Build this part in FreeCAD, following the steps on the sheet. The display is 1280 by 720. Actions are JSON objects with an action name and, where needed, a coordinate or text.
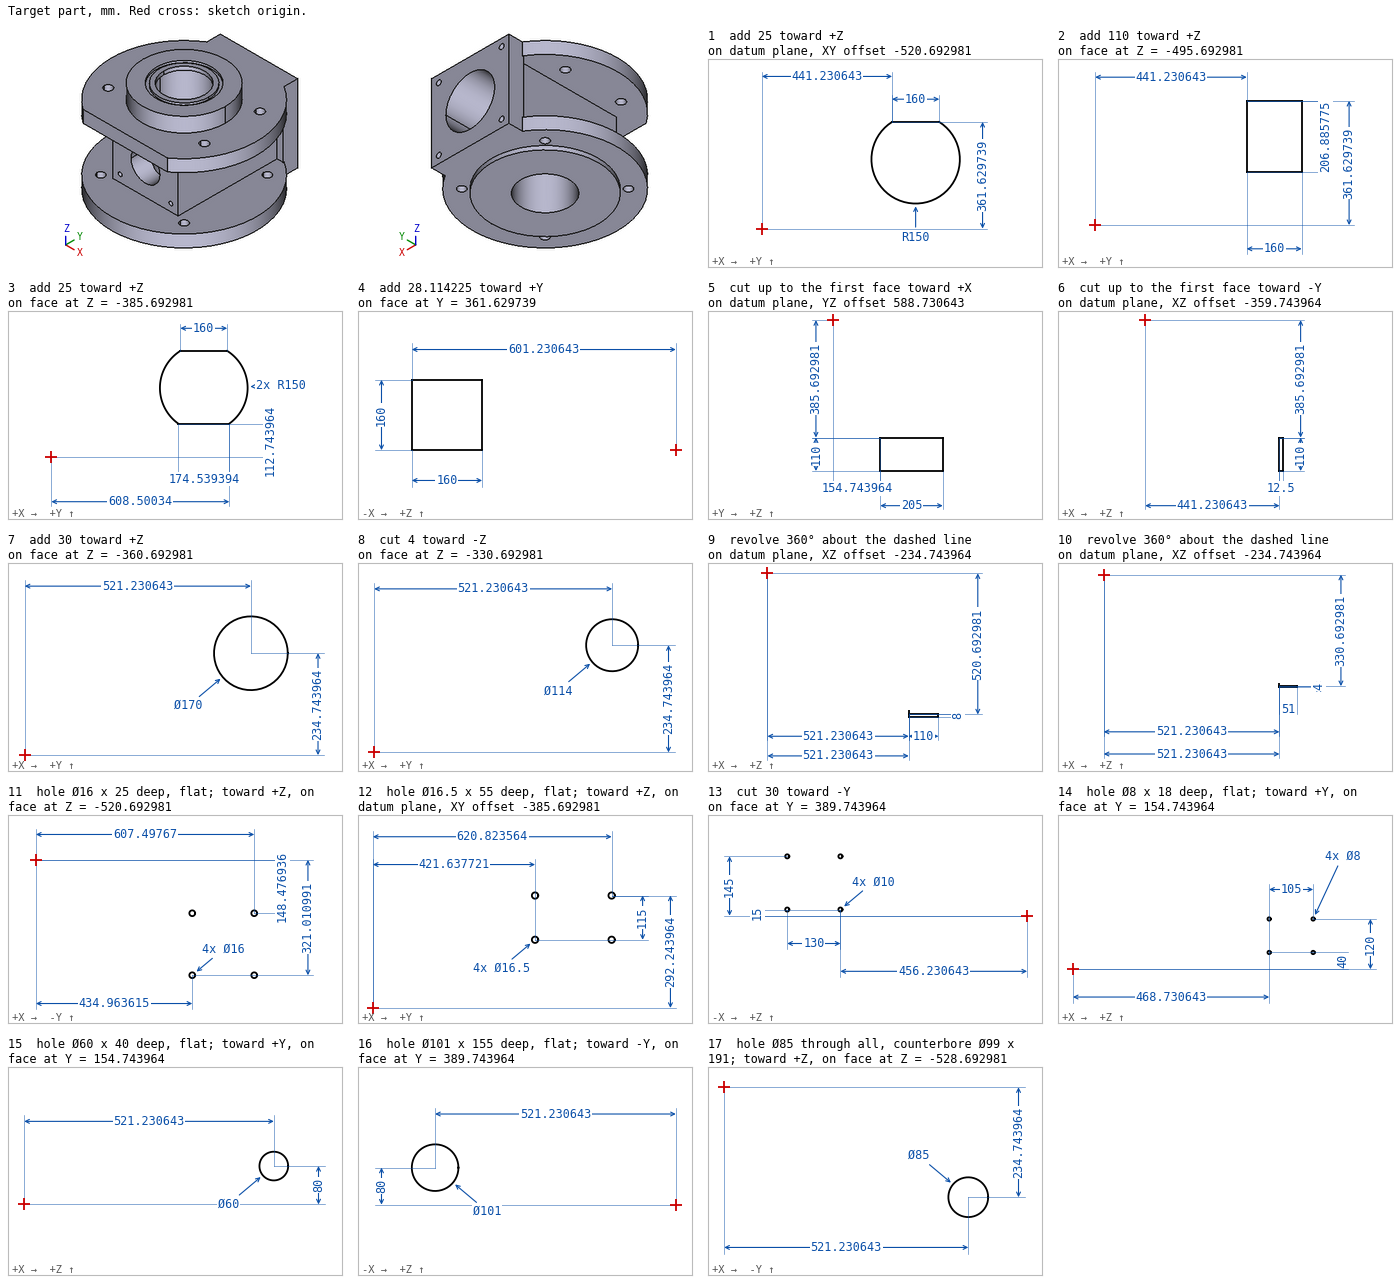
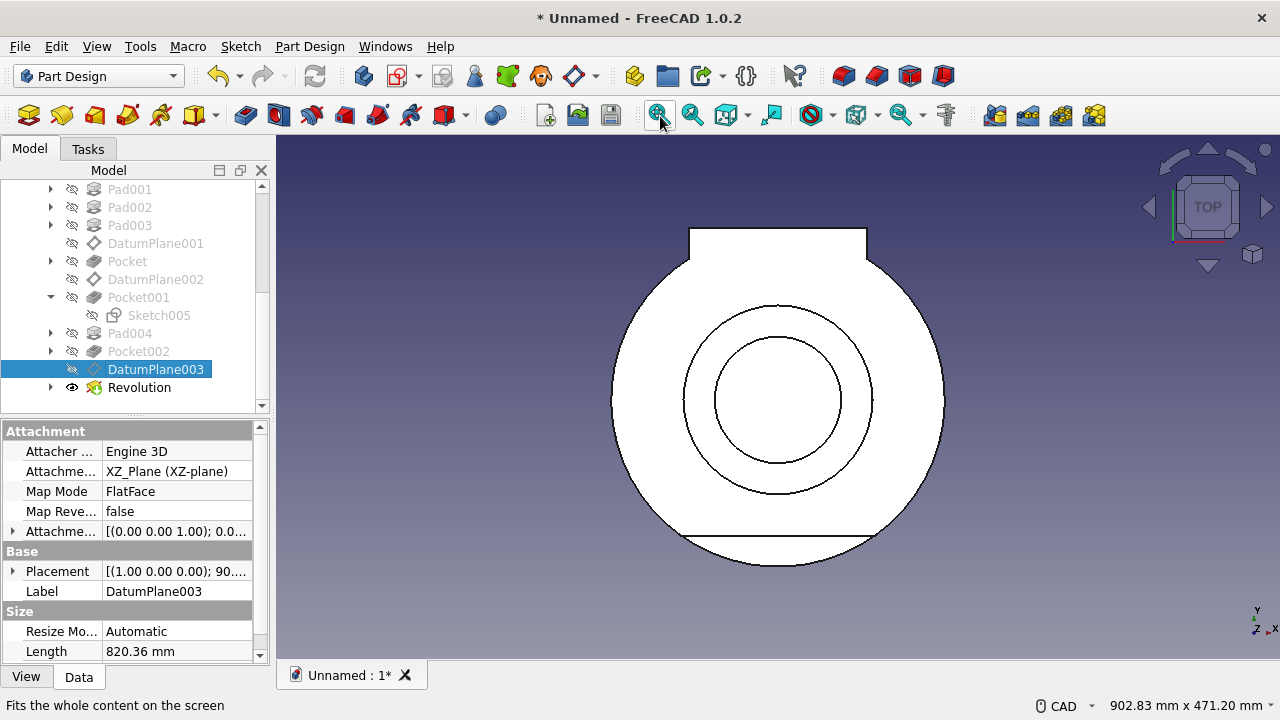
{"action": "scroll", "coordinate": [141, 293], "scroll_direction": "down", "scroll_amount": 3}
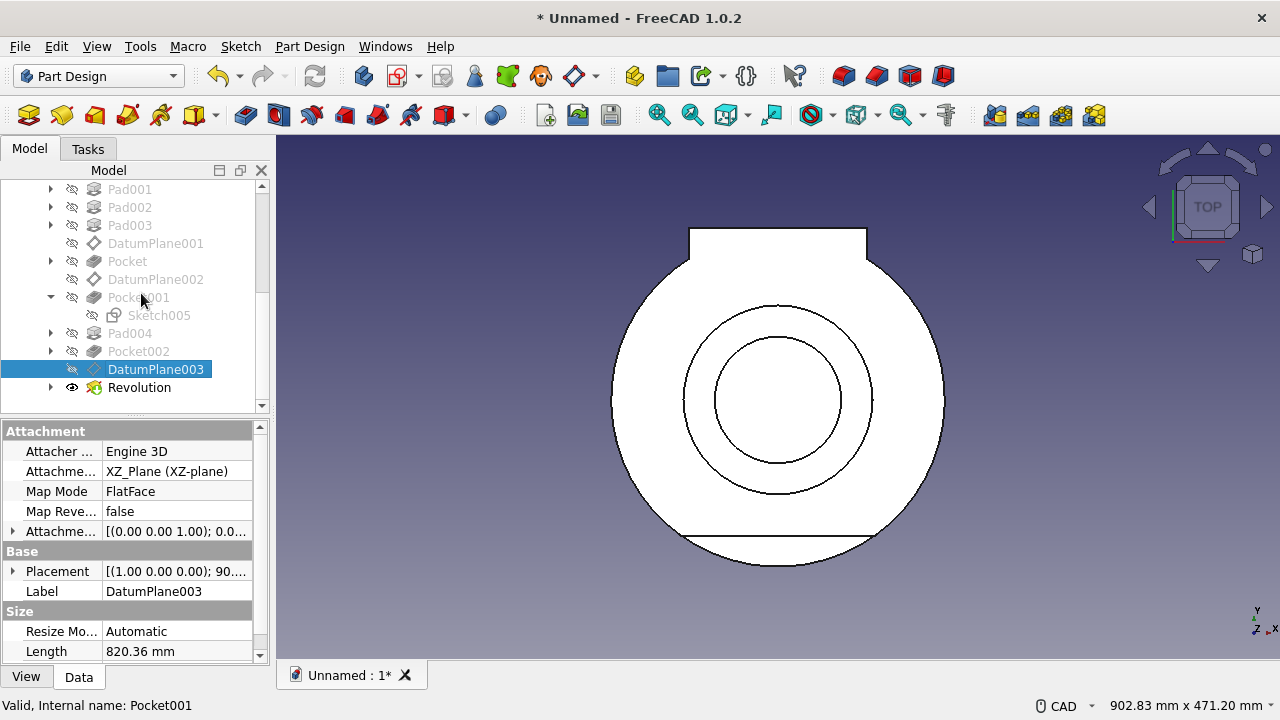
{"action": "scroll", "coordinate": [141, 293], "scroll_direction": "up", "scroll_amount": 15}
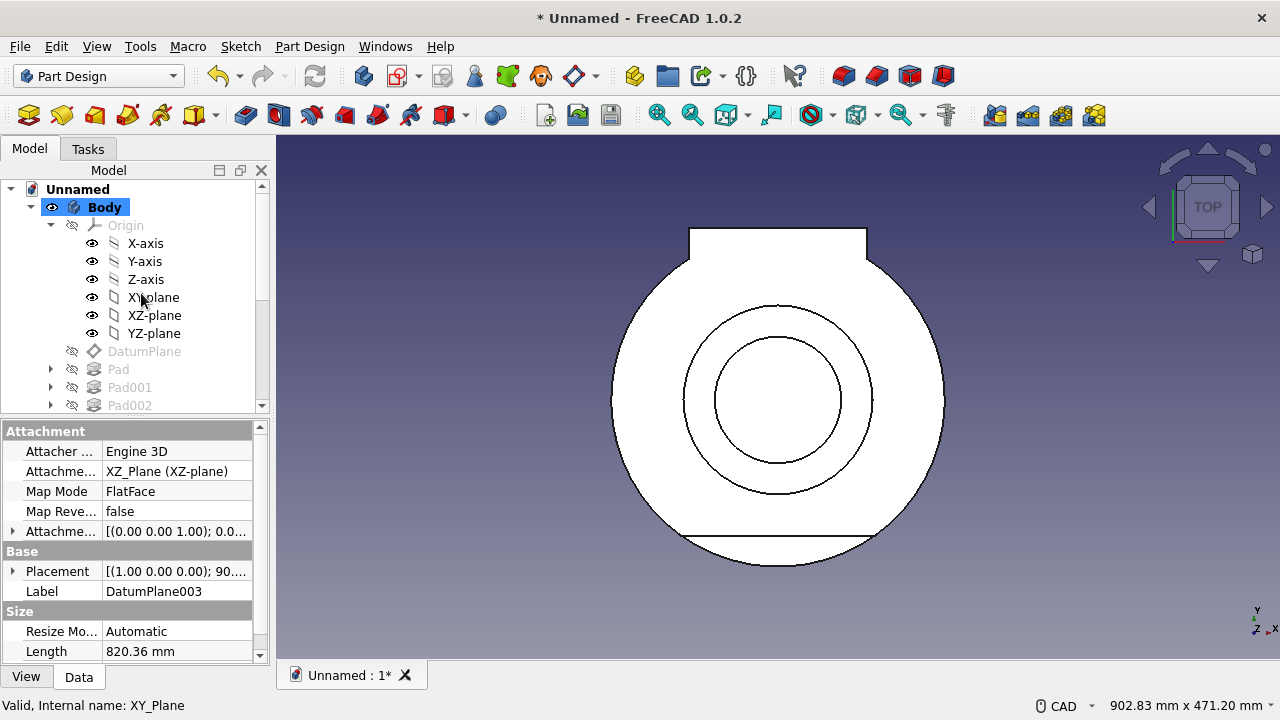
{"action": "left_click", "coordinate": [137, 315]}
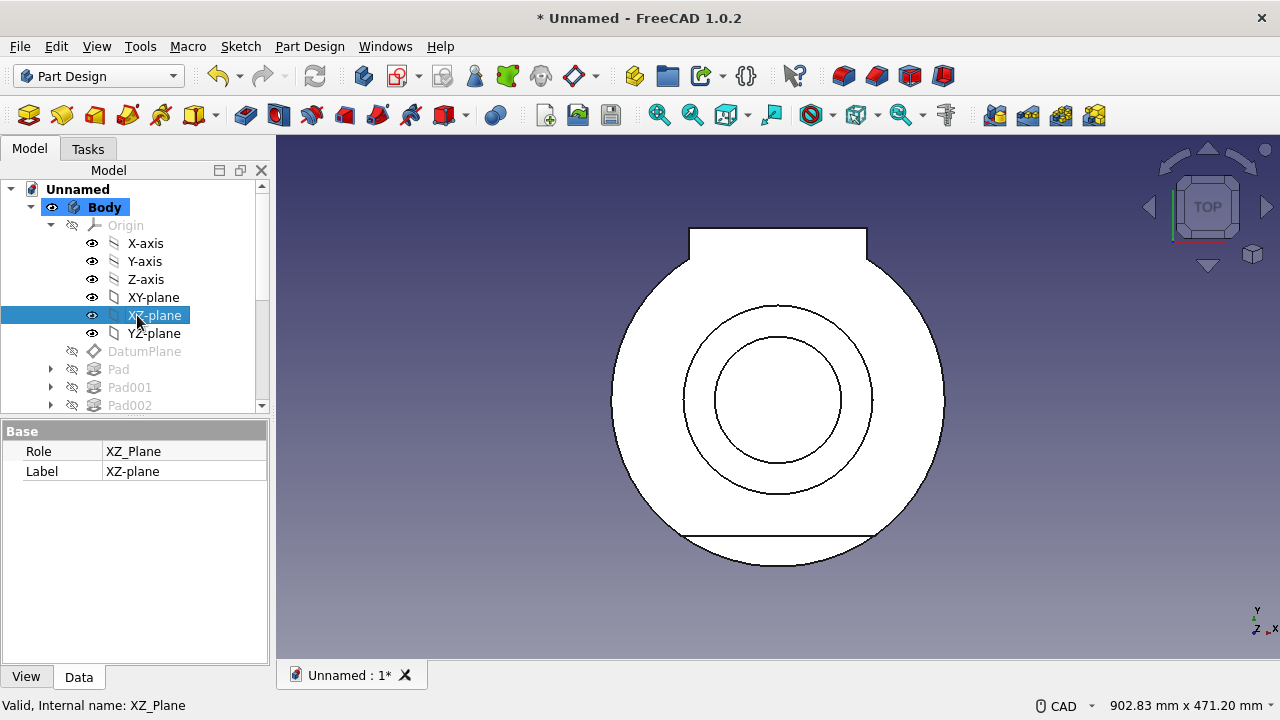
{"action": "left_click", "coordinate": [574, 76]}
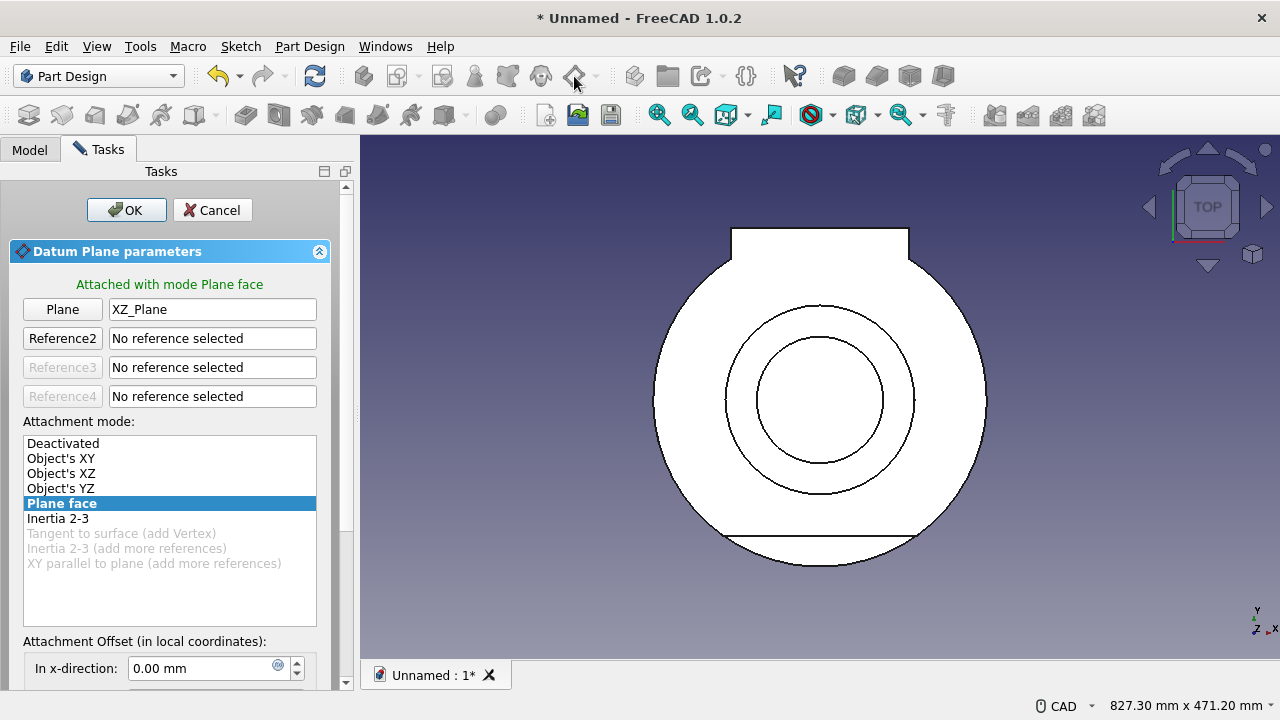
{"action": "scroll", "coordinate": [346, 436], "scroll_direction": "down", "scroll_amount": 2}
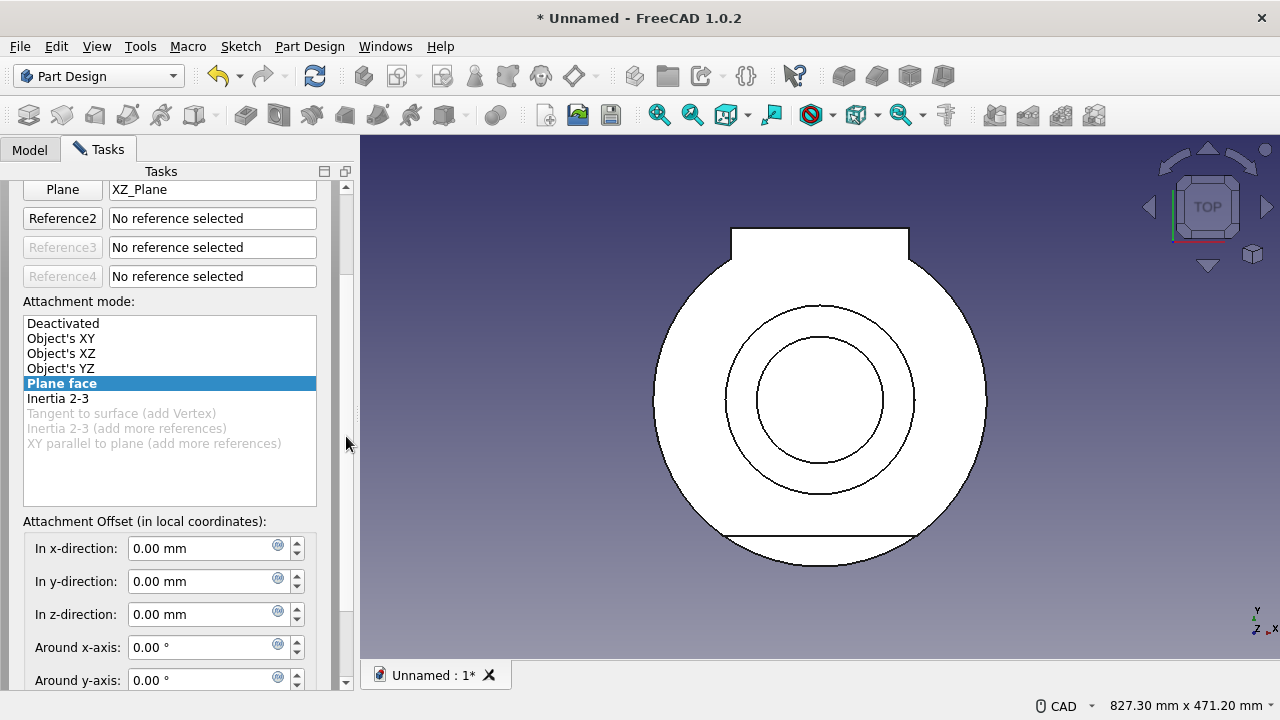
{"action": "triple_click", "coordinate": [210, 614]}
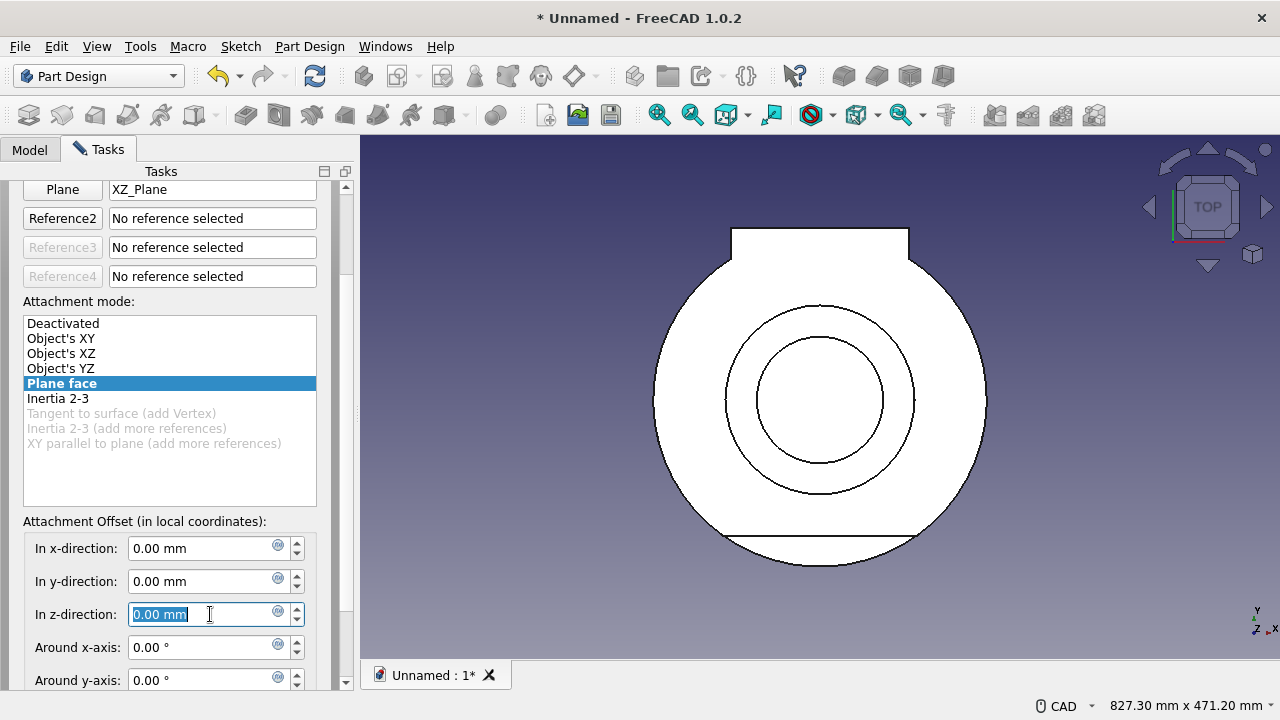
{"action": "type", "text": "-234.743964"}
{"action": "key", "text": "Tab"}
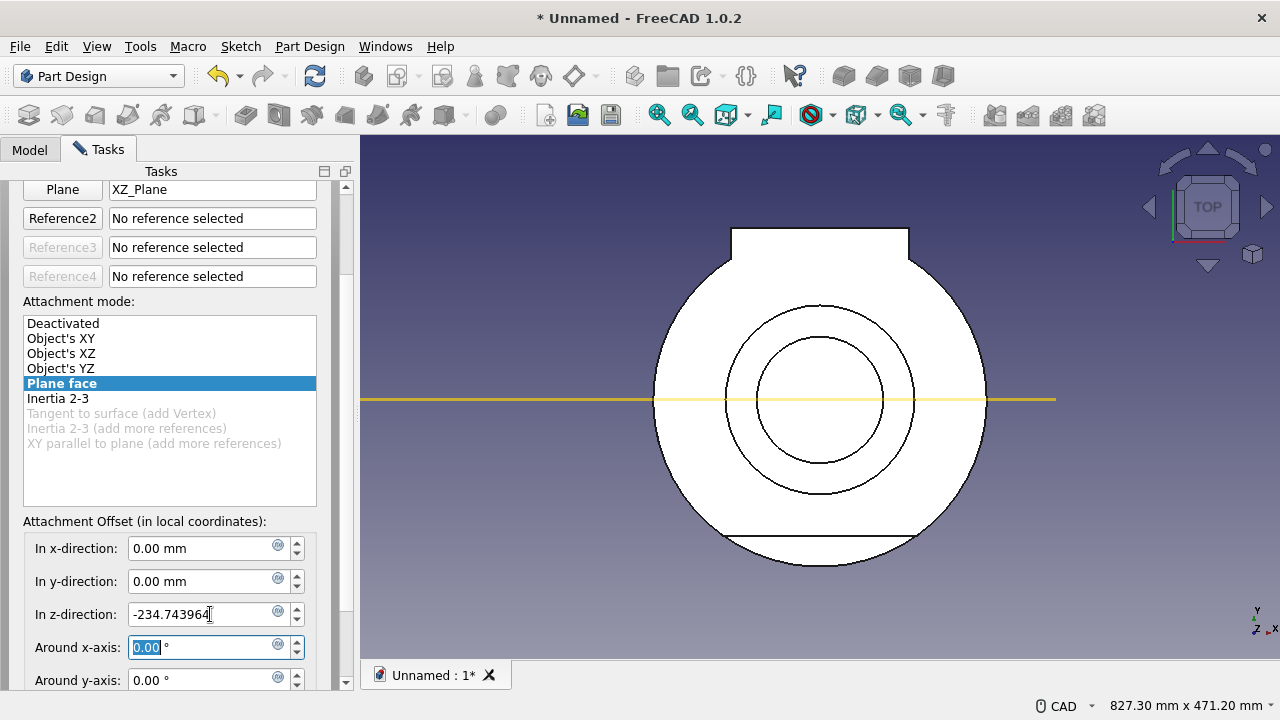
{"action": "scroll", "coordinate": [346, 436], "scroll_direction": "up", "scroll_amount": 3}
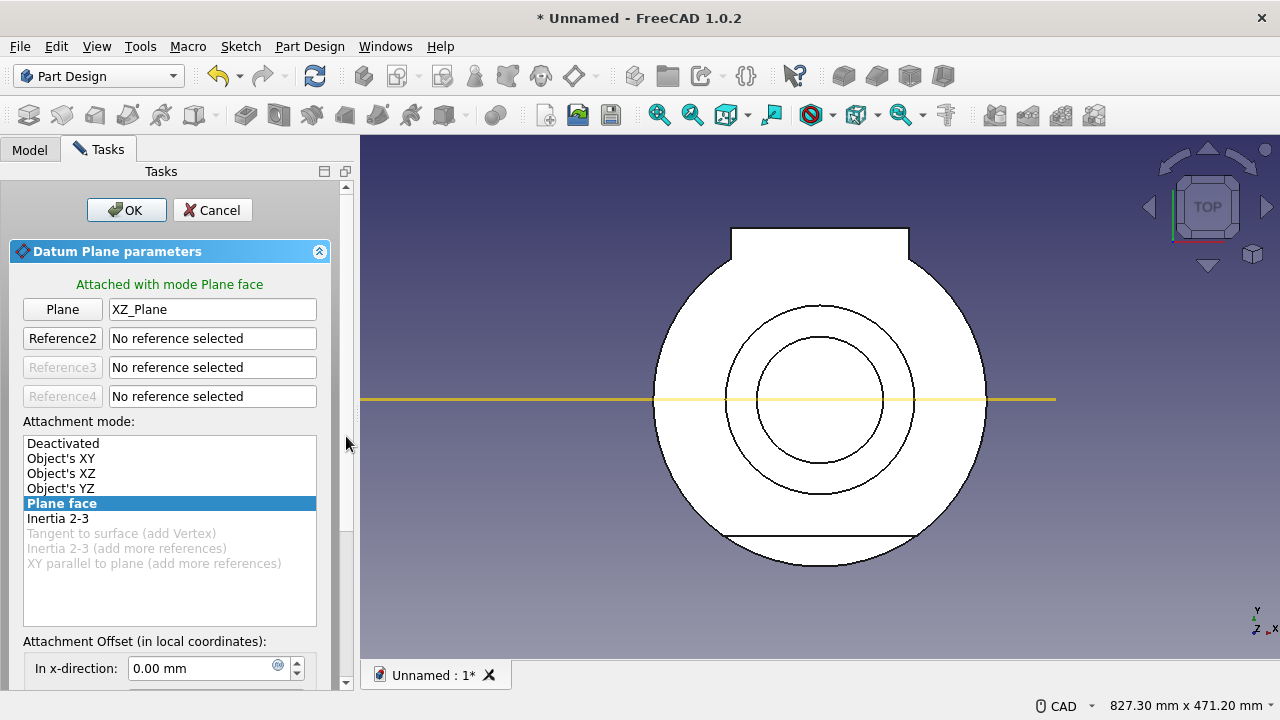
{"action": "left_click", "coordinate": [127, 210]}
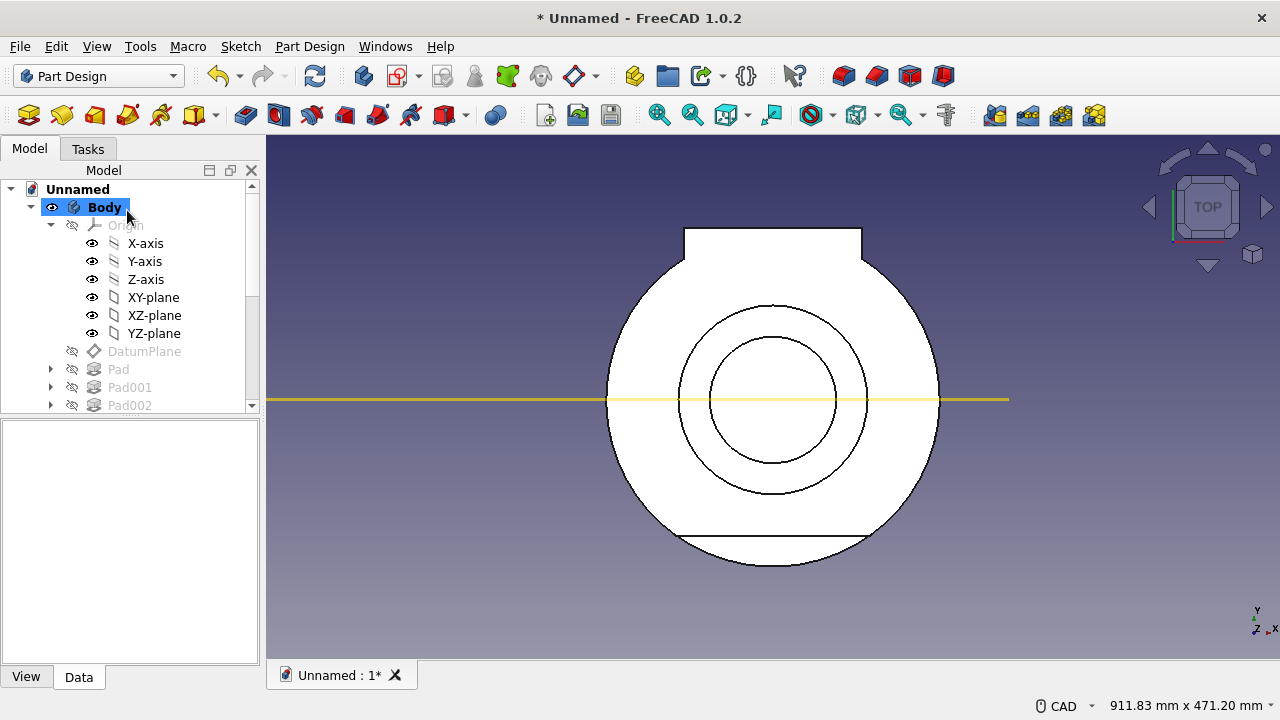
{"action": "scroll", "coordinate": [101, 293], "scroll_direction": "down", "scroll_amount": 3}